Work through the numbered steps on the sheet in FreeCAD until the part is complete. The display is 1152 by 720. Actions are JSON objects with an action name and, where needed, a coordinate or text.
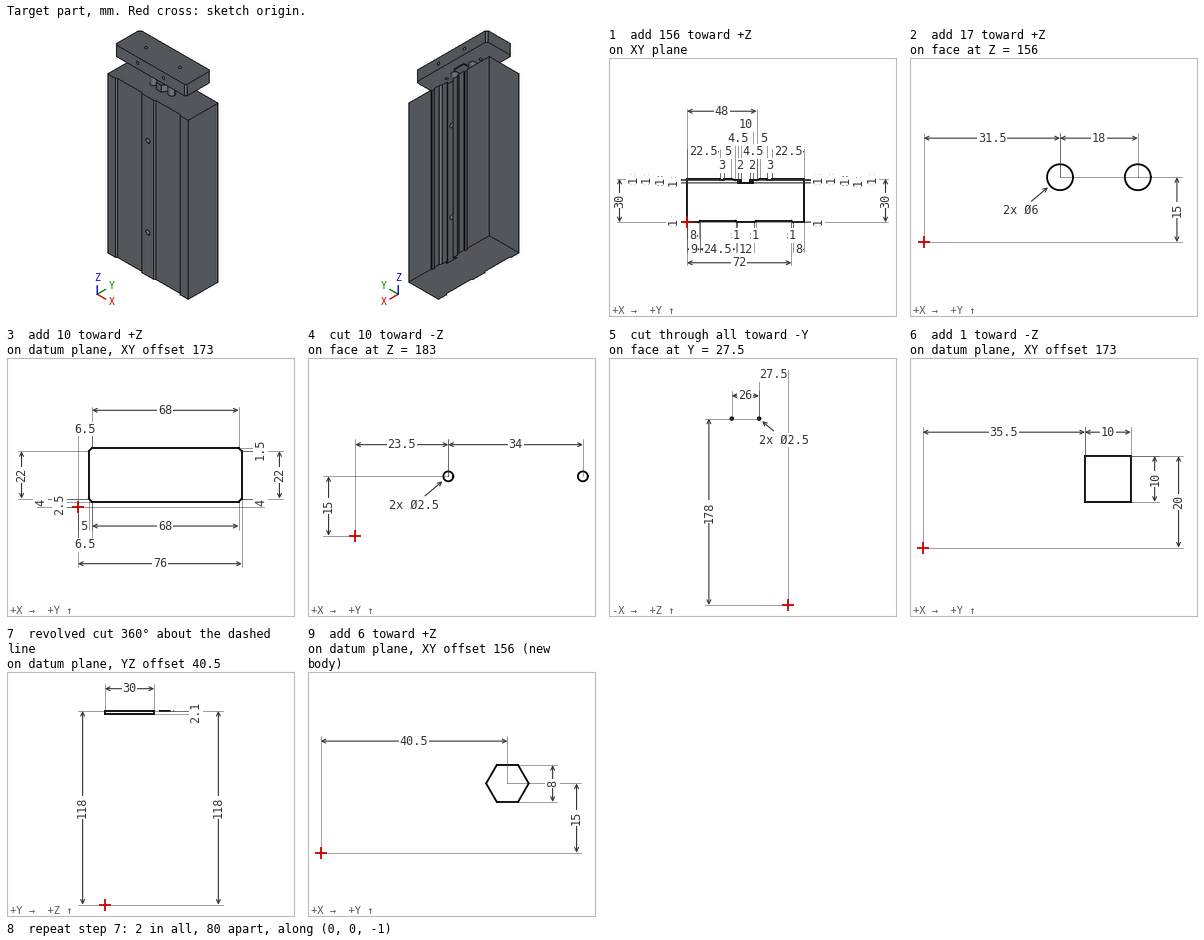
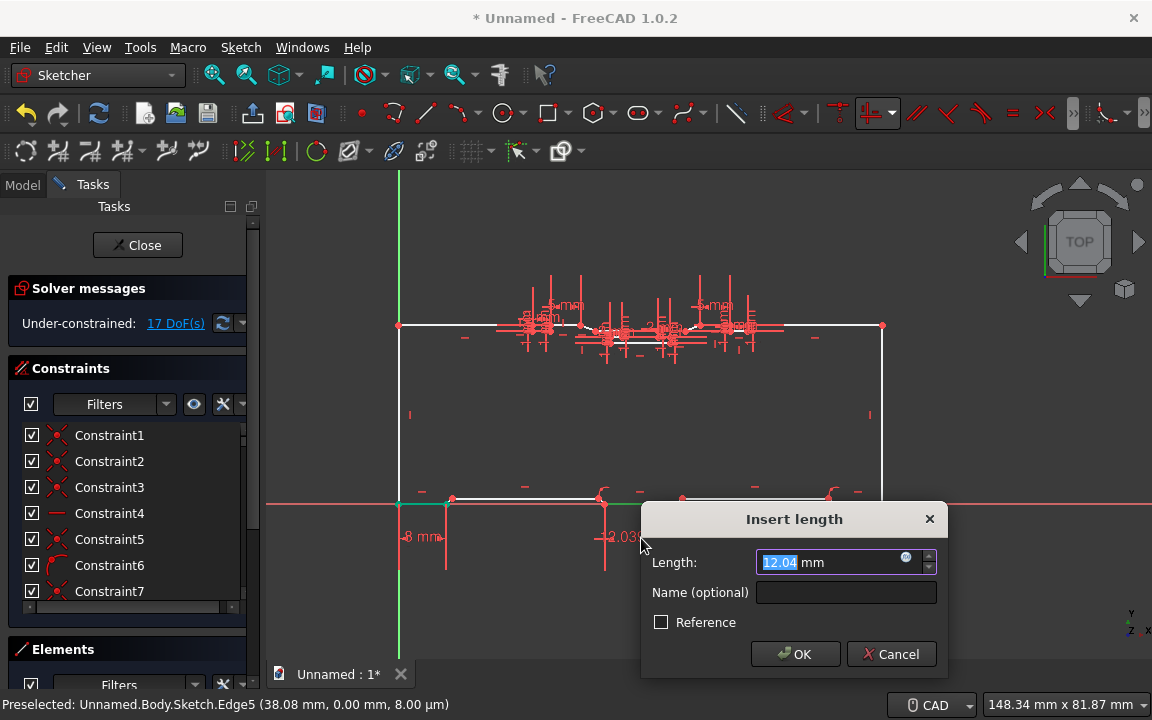
{"action": "type", "text": "12"}
{"action": "key", "text": "Return"}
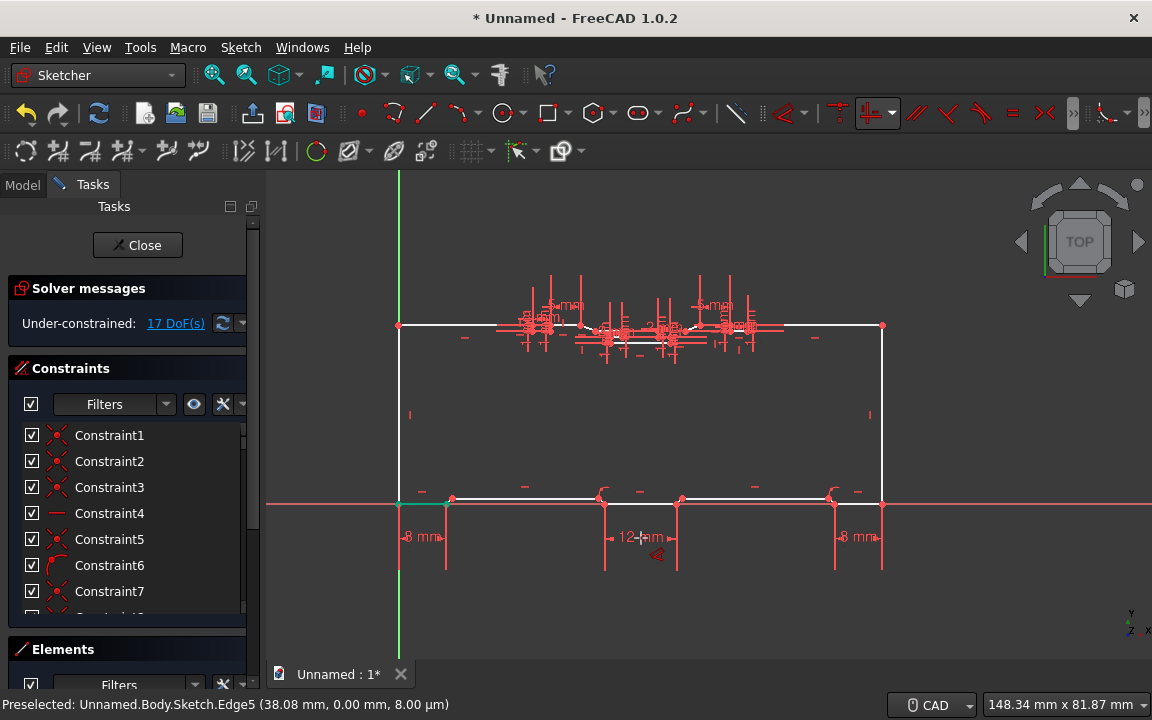
{"action": "left_click", "coordinate": [882, 450]}
{"action": "left_click", "coordinate": [916, 415]}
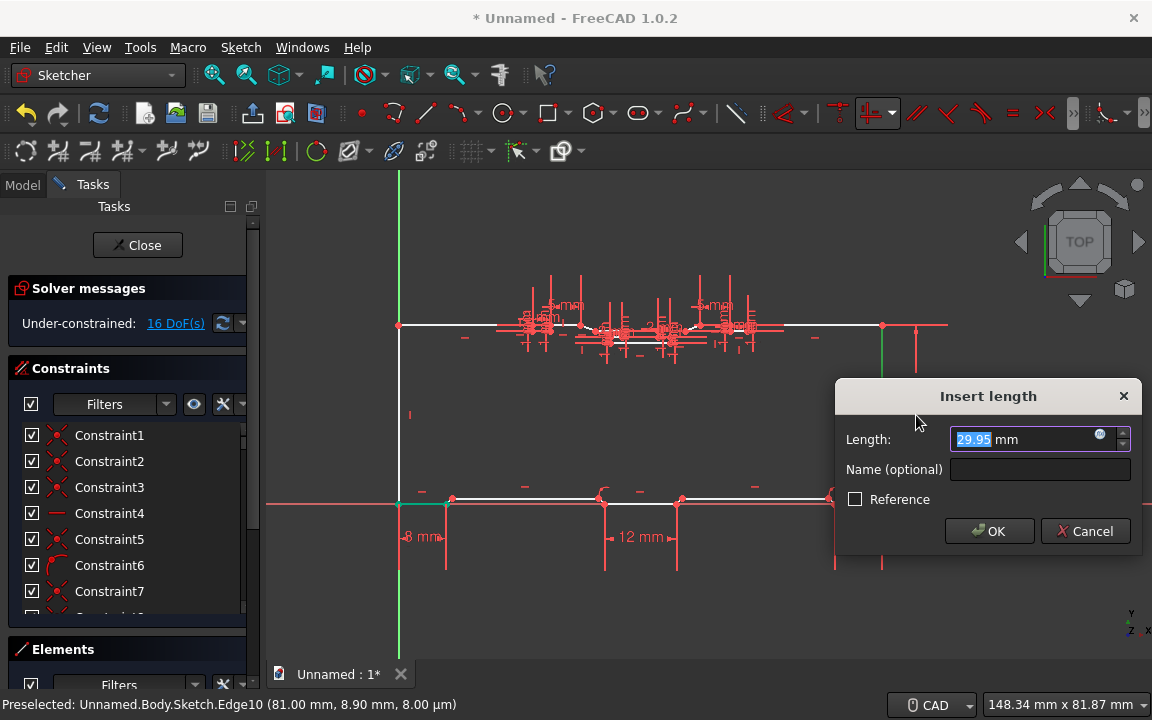
{"action": "type", "text": "30"}
{"action": "key", "text": "Return"}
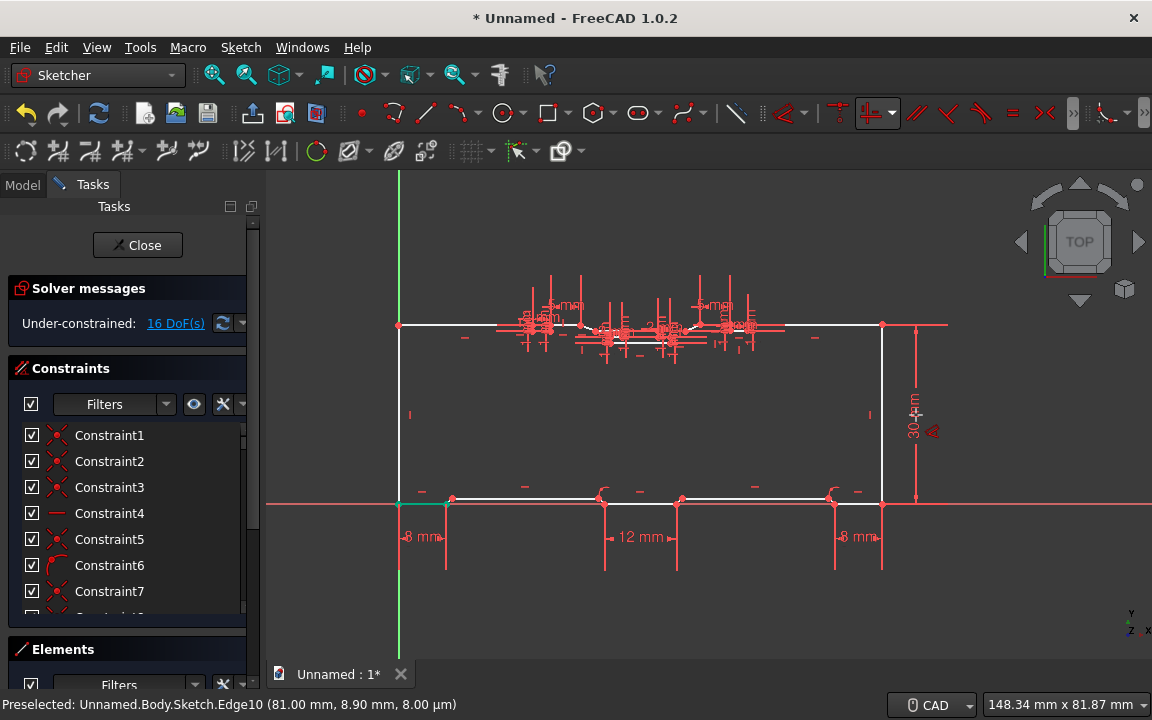
{"action": "left_click", "coordinate": [646, 343]}
{"action": "left_click", "coordinate": [640, 309]}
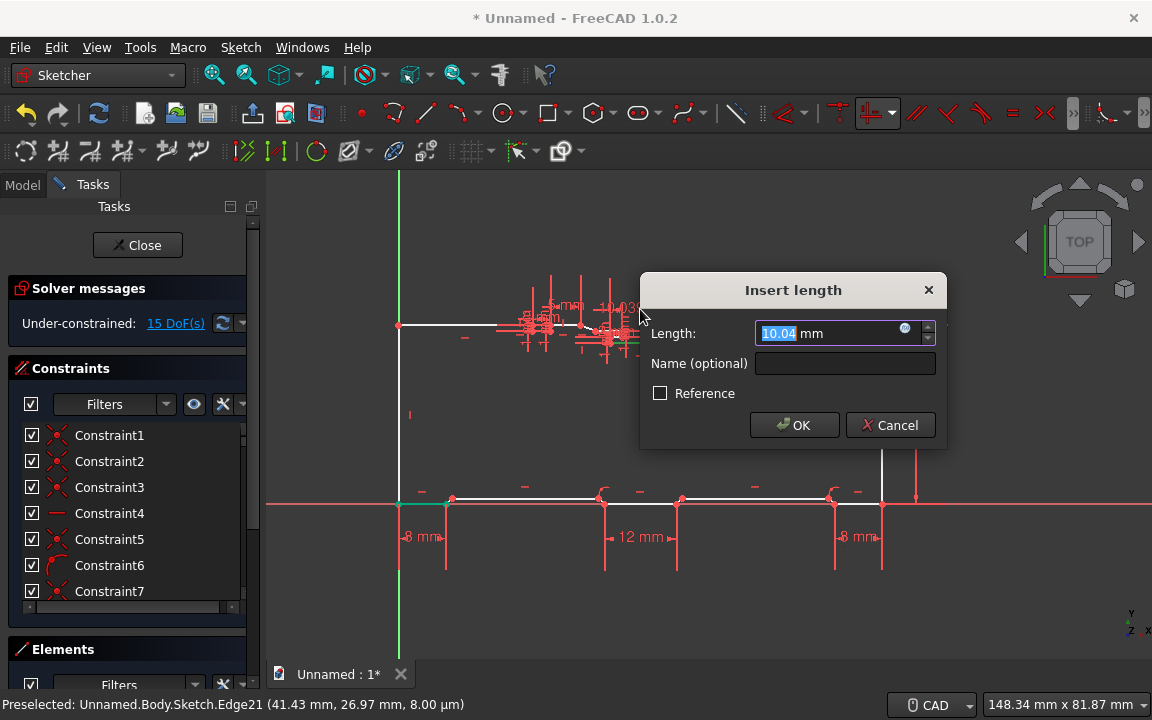
{"action": "type", "text": "10"}
{"action": "key", "text": "Return"}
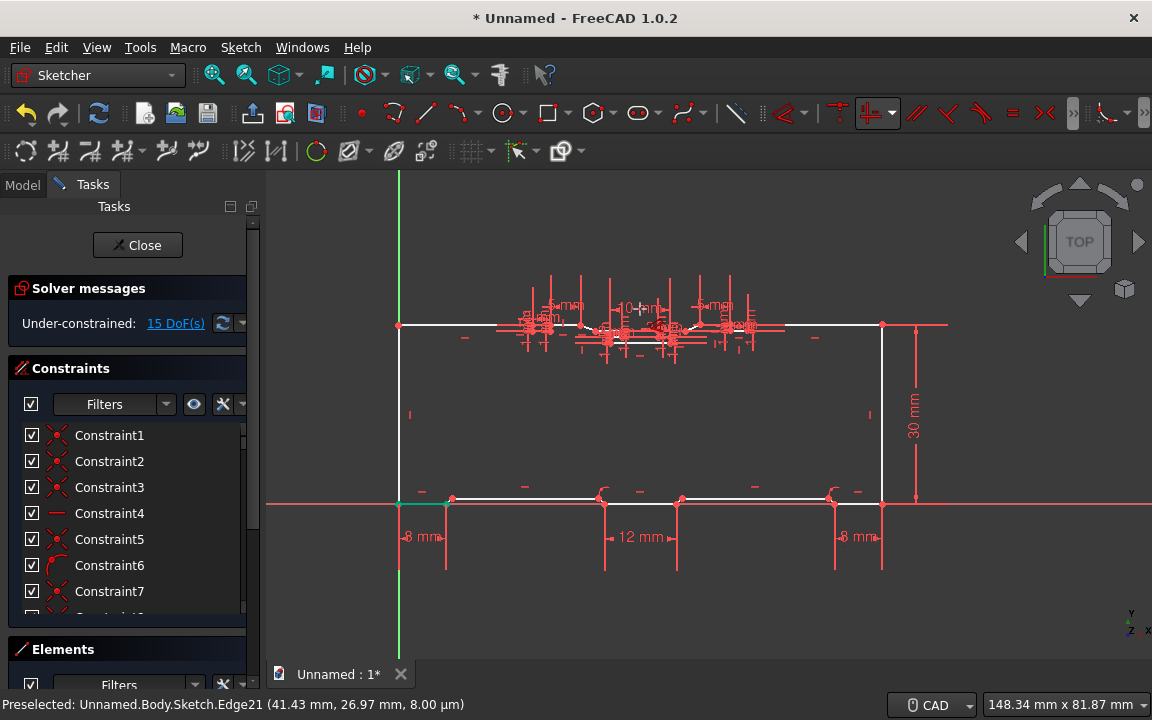
{"action": "left_click", "coordinate": [399, 379]}
{"action": "left_click", "coordinate": [365, 415]}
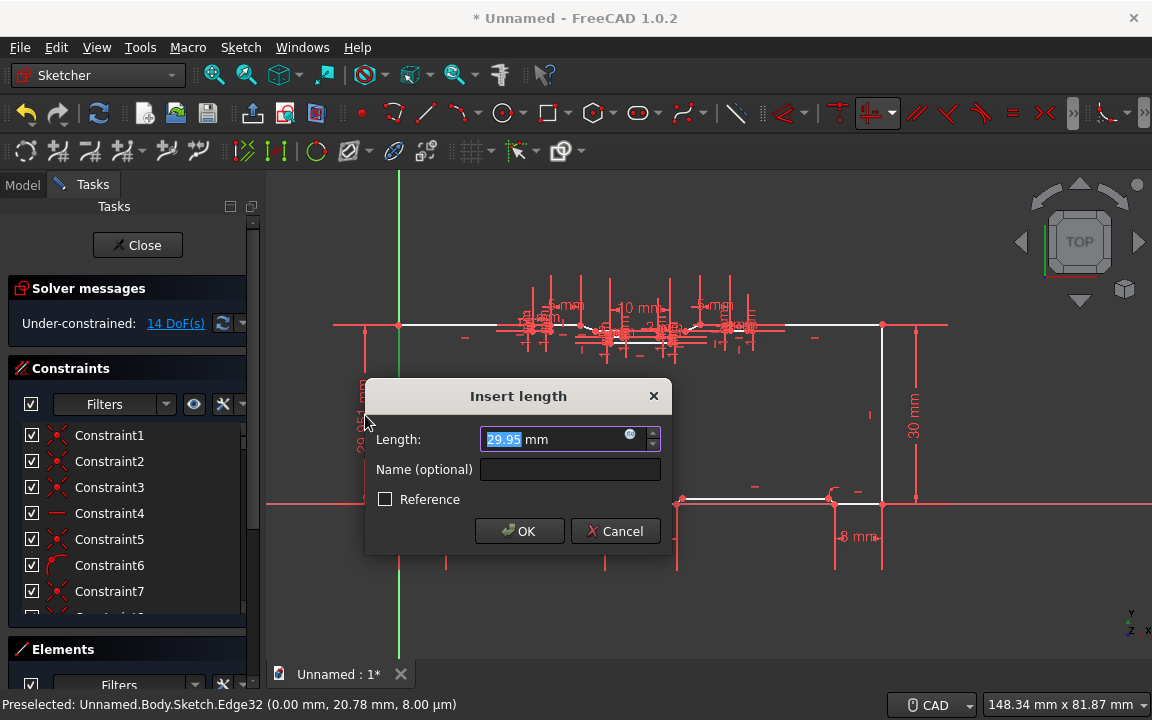
{"action": "type", "text": "30"}
{"action": "key", "text": "Return"}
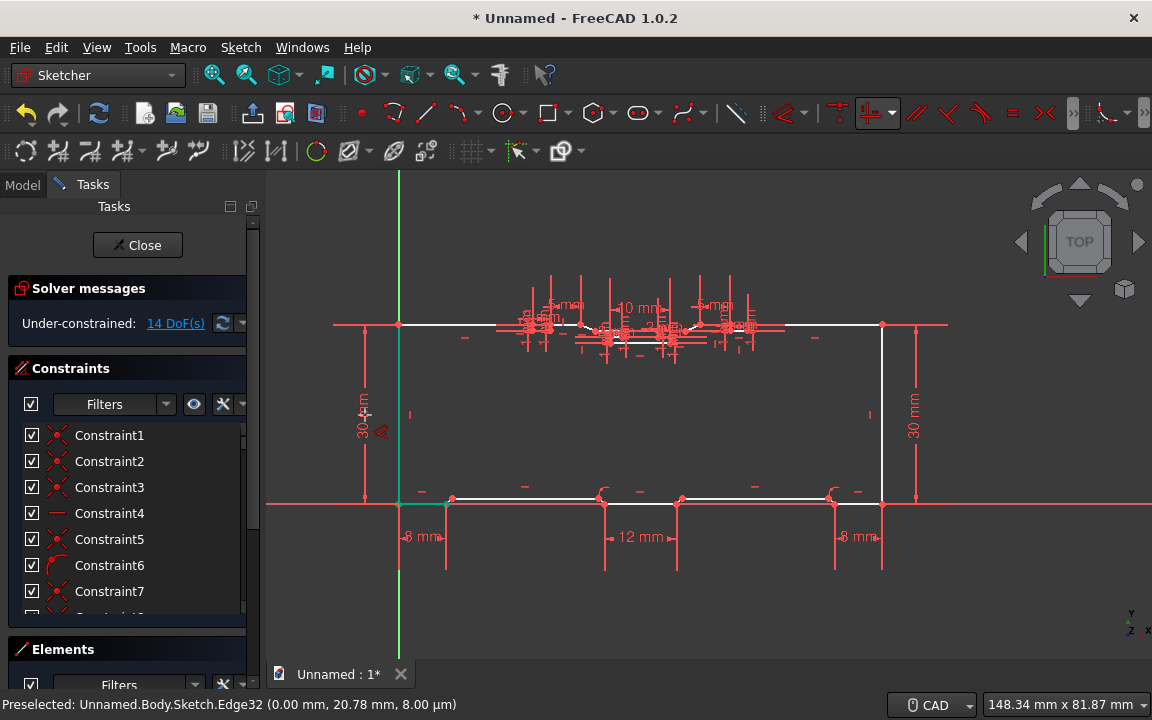
{"action": "scroll", "coordinate": [452, 499], "scroll_direction": "up", "scroll_amount": 3}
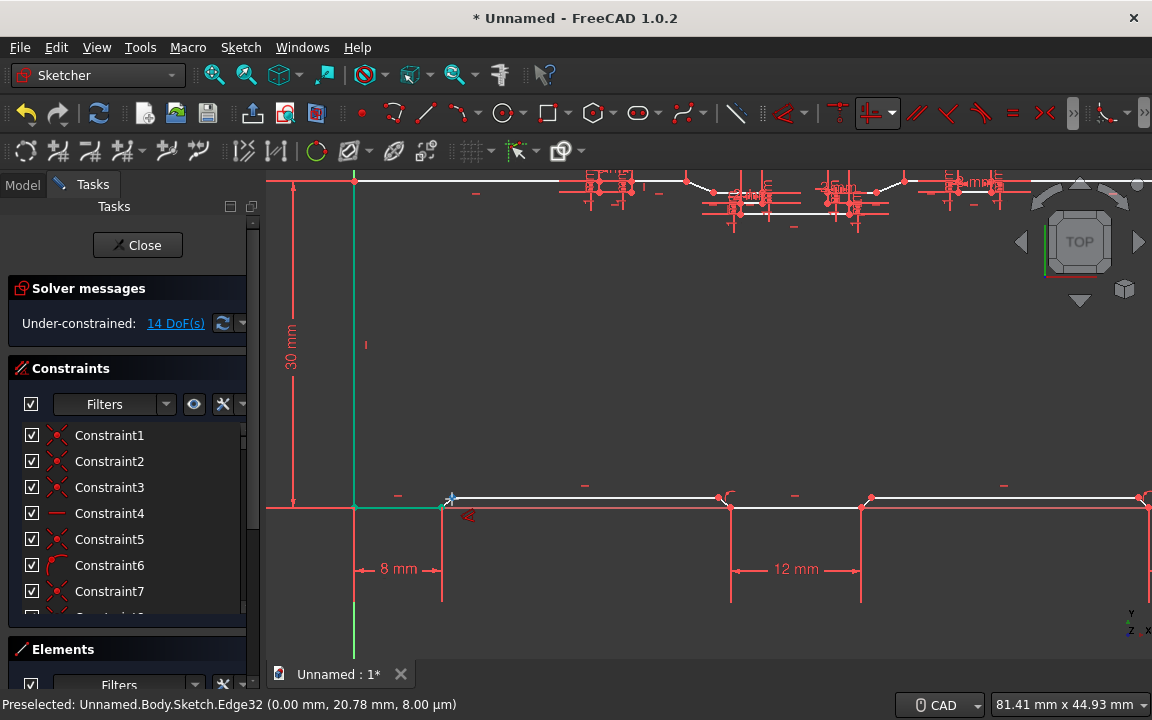
{"action": "left_click", "coordinate": [453, 498]}
{"action": "left_click", "coordinate": [404, 542]}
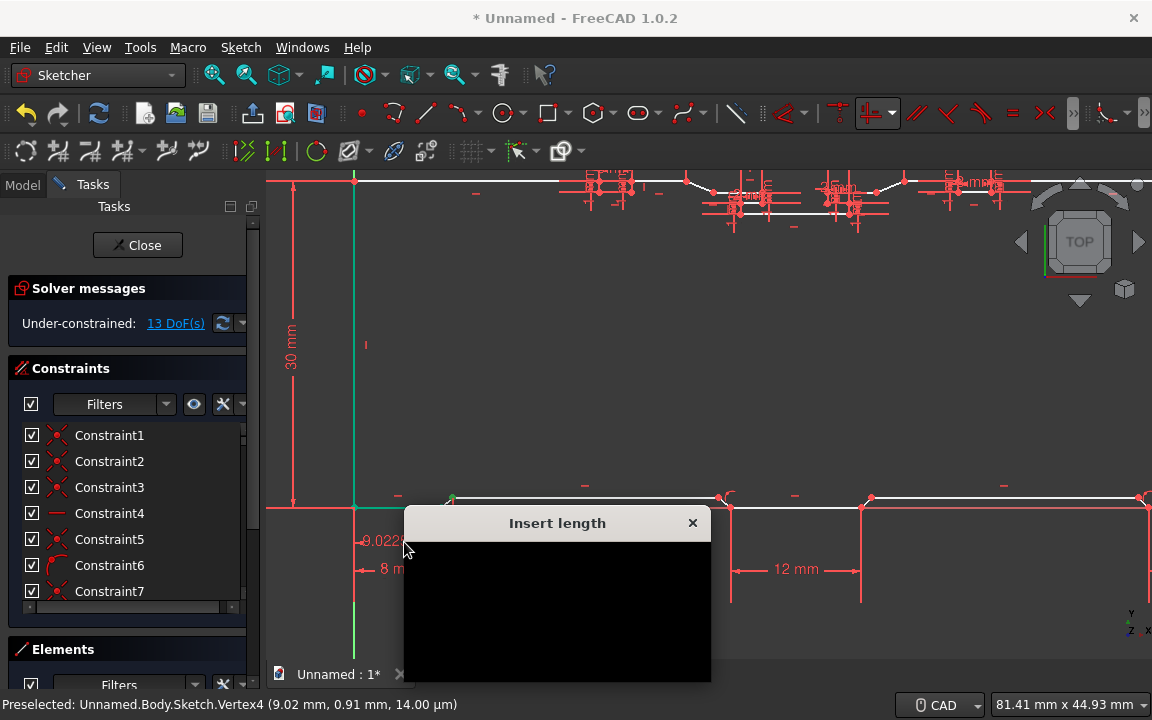
{"action": "type", "text": "9"}
{"action": "key", "text": "Return"}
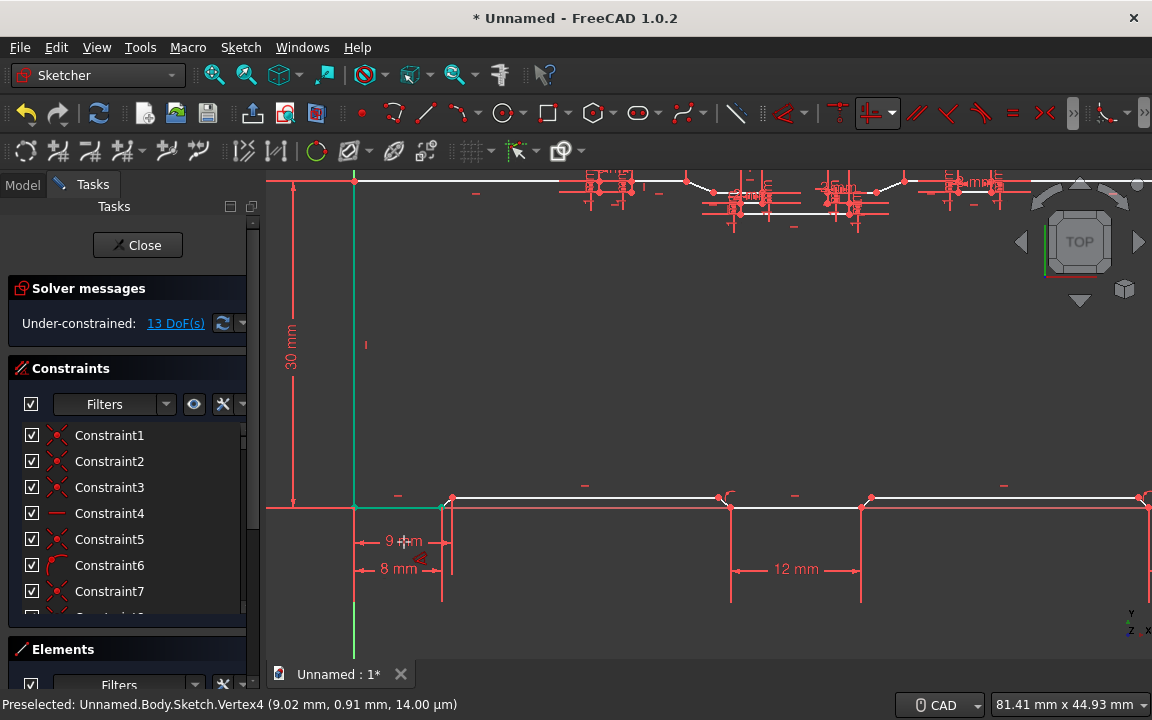
{"action": "scroll", "coordinate": [452, 498], "scroll_direction": "up", "scroll_amount": 7}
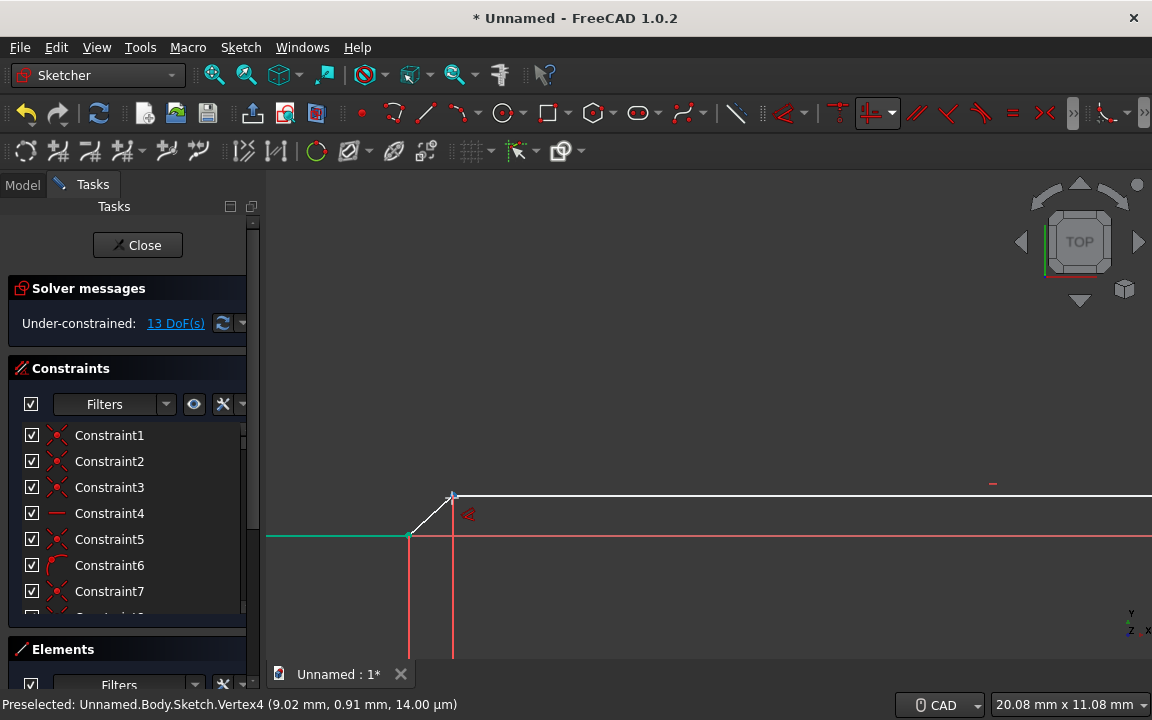
{"action": "left_click", "coordinate": [453, 496]}
{"action": "left_click", "coordinate": [487, 516]}